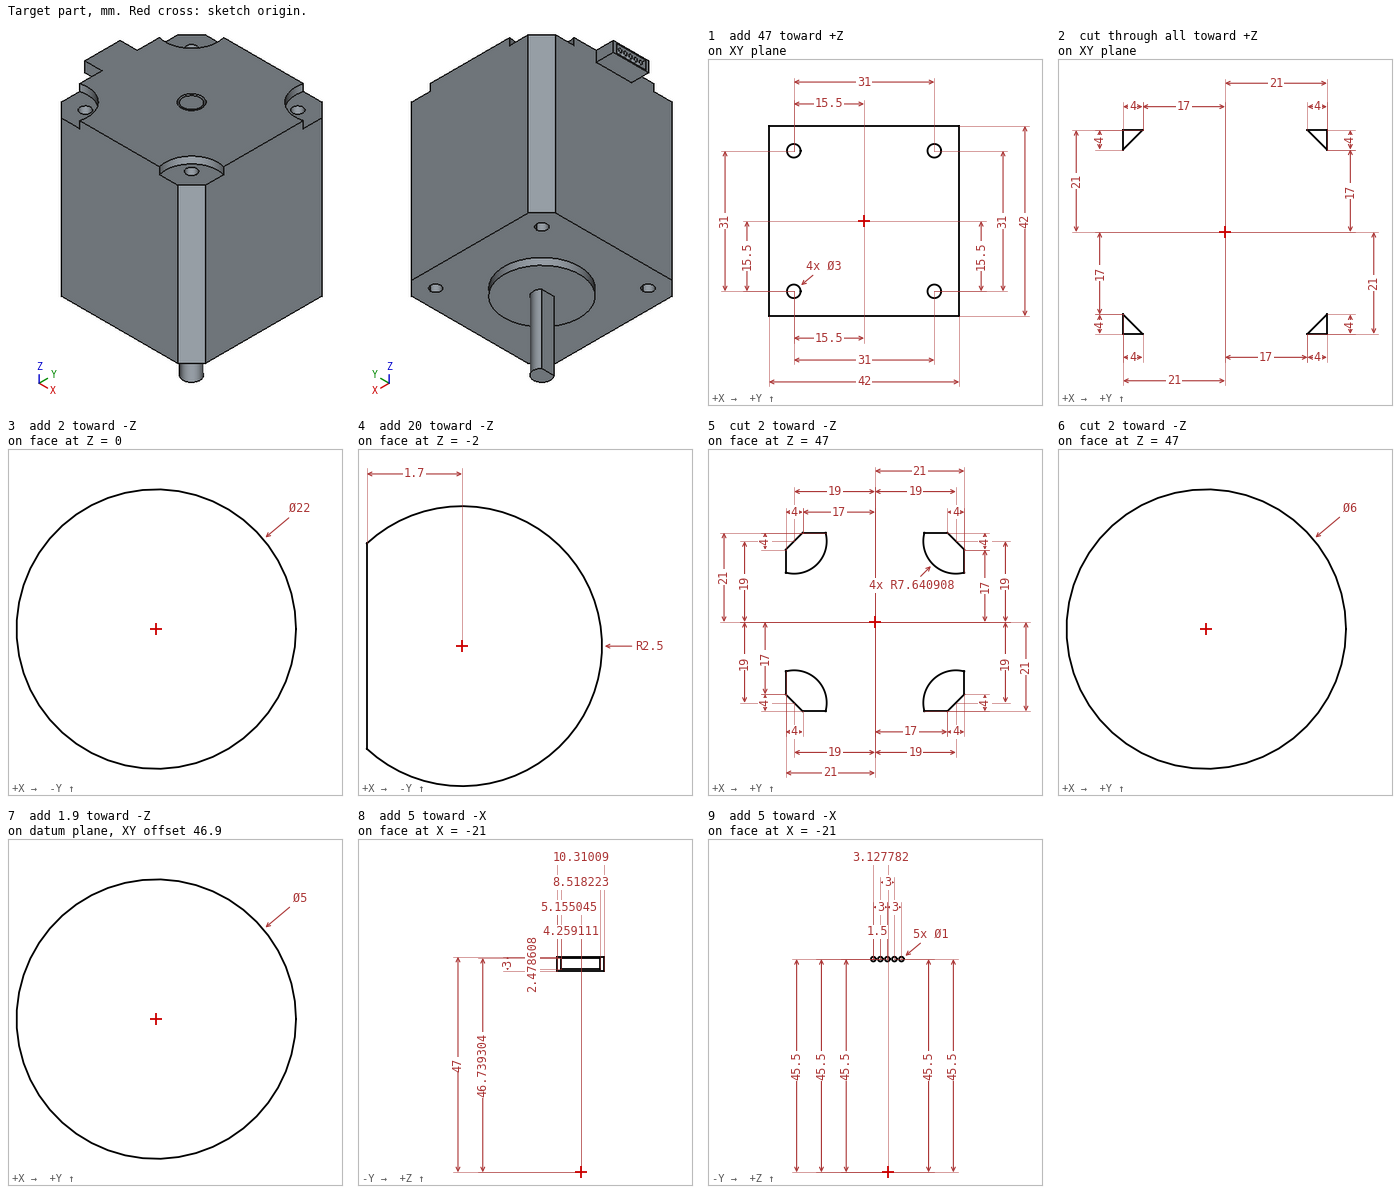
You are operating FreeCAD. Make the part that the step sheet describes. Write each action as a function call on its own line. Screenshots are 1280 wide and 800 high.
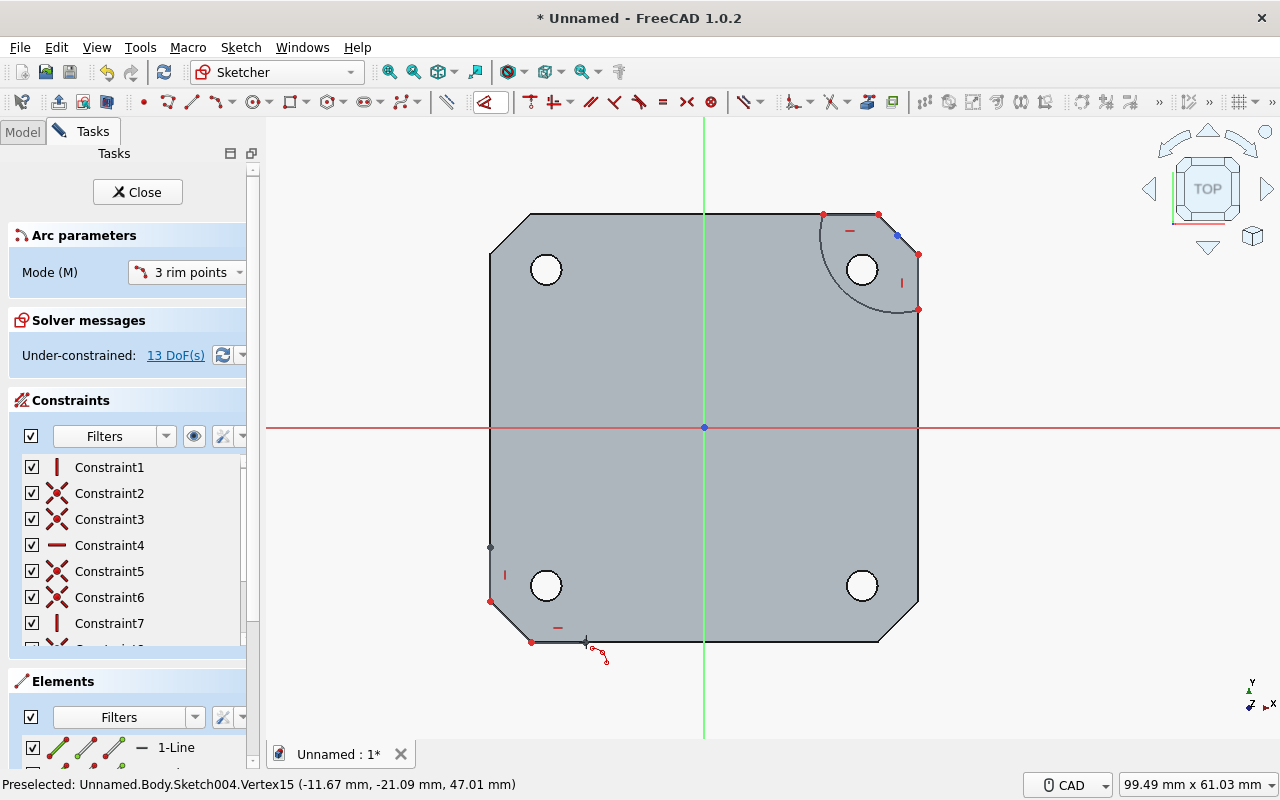
click(585, 643)
click(490, 547)
click(566, 566)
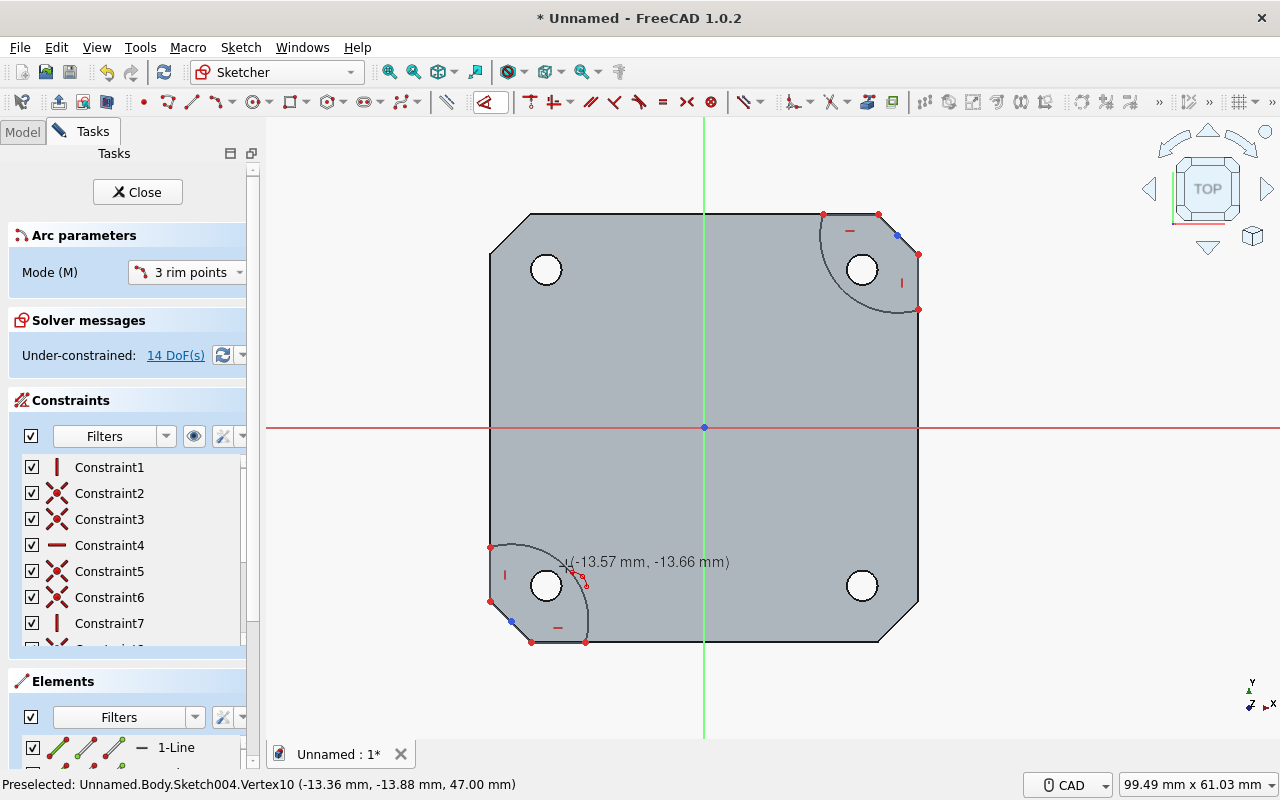
click(168, 102)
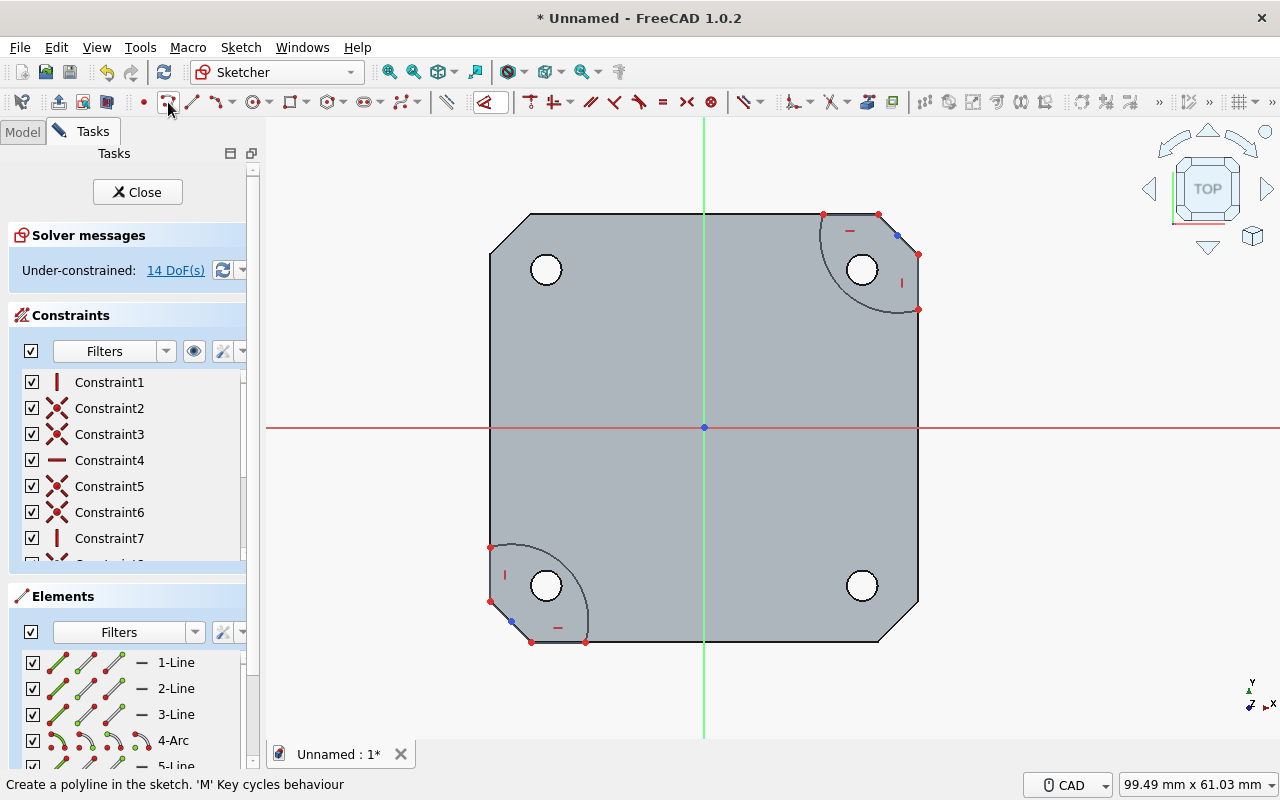
click(586, 214)
click(531, 214)
click(490, 254)
click(490, 309)
right_click(490, 309)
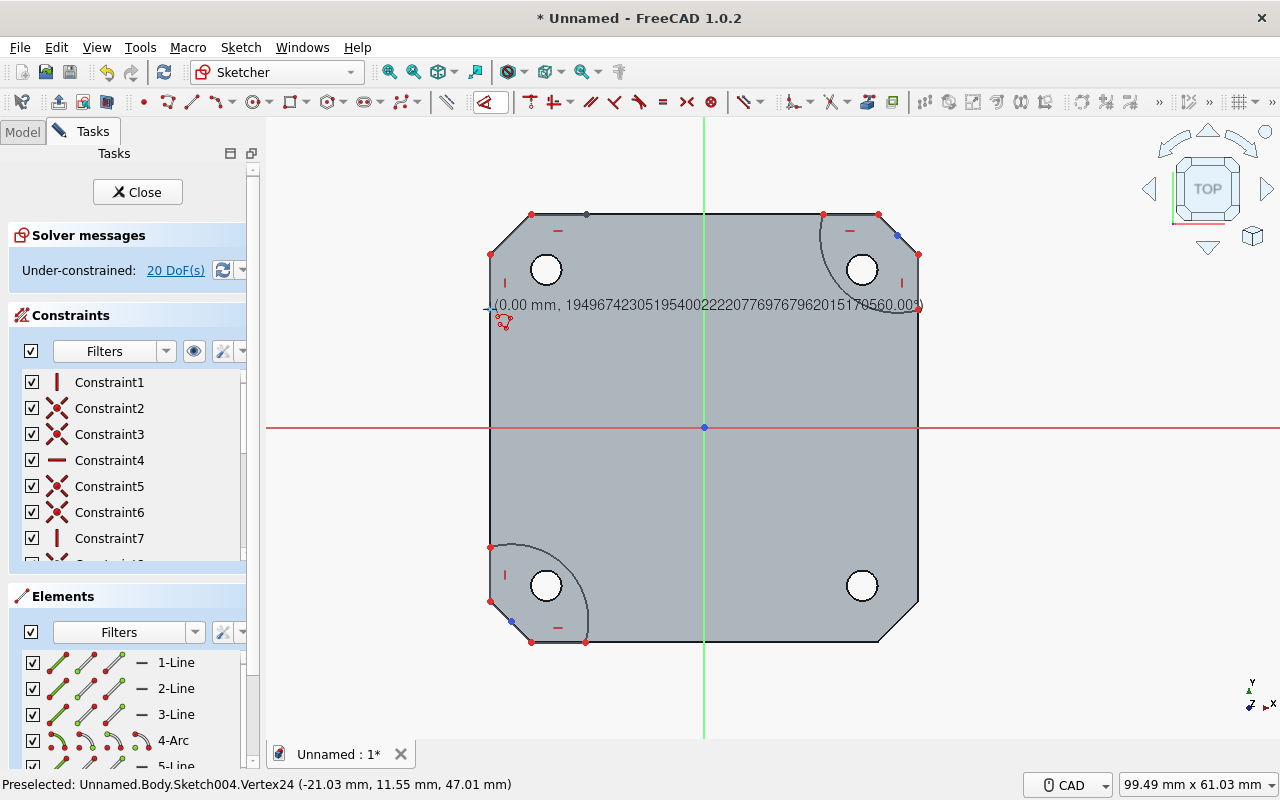
click(216, 102)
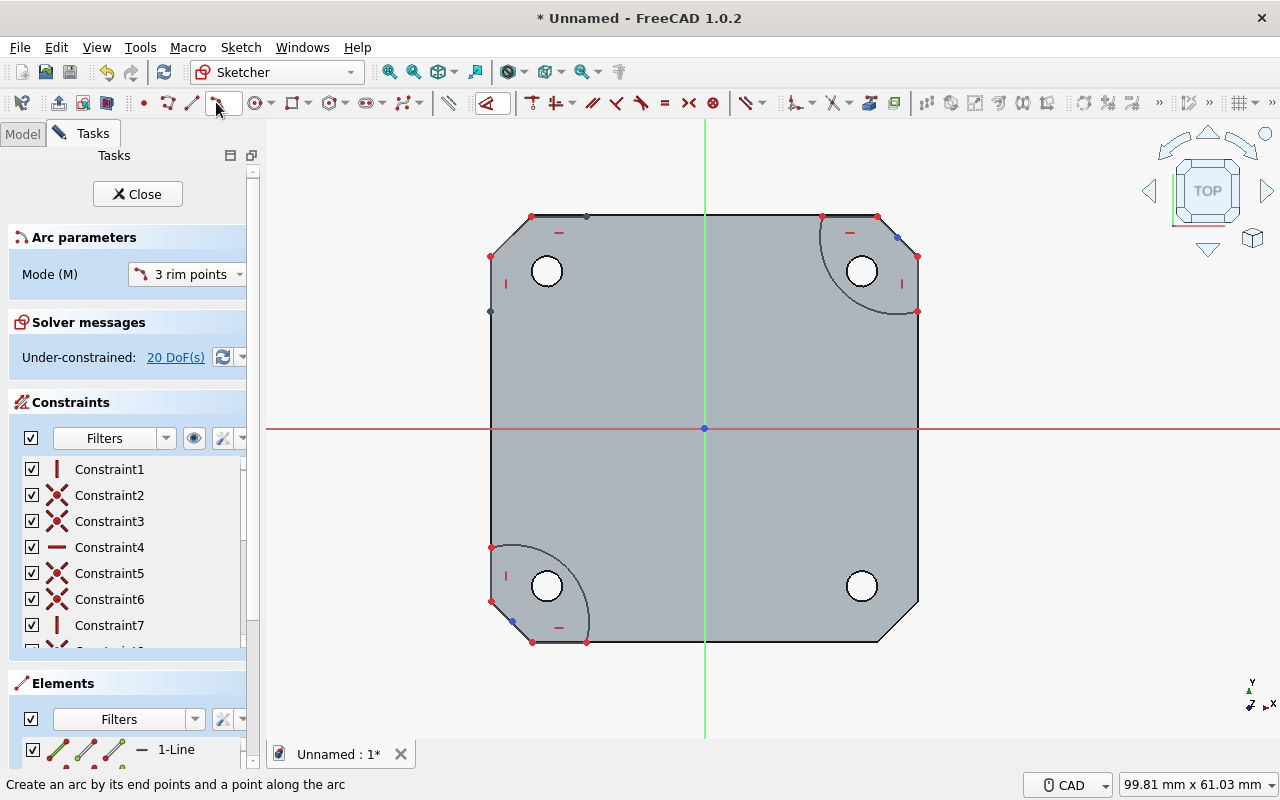
click(491, 311)
click(587, 217)
click(566, 291)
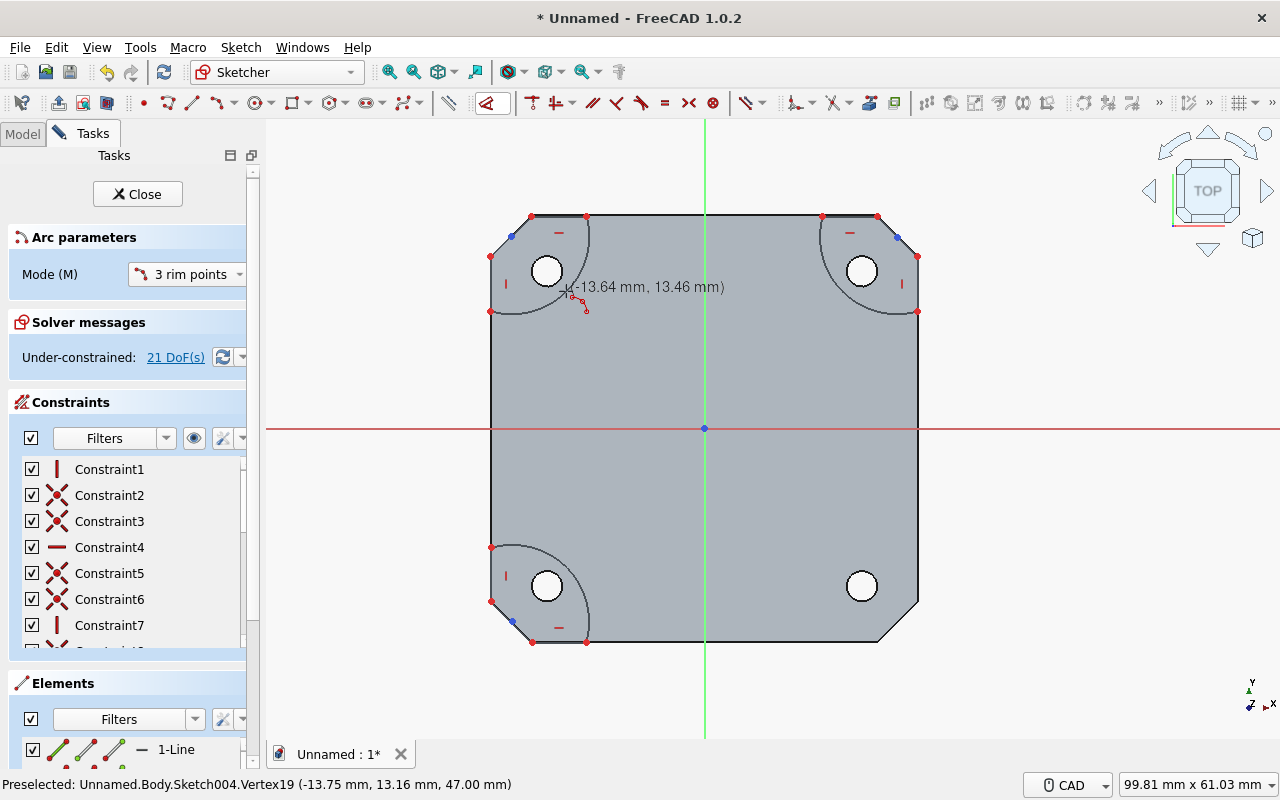
click(168, 104)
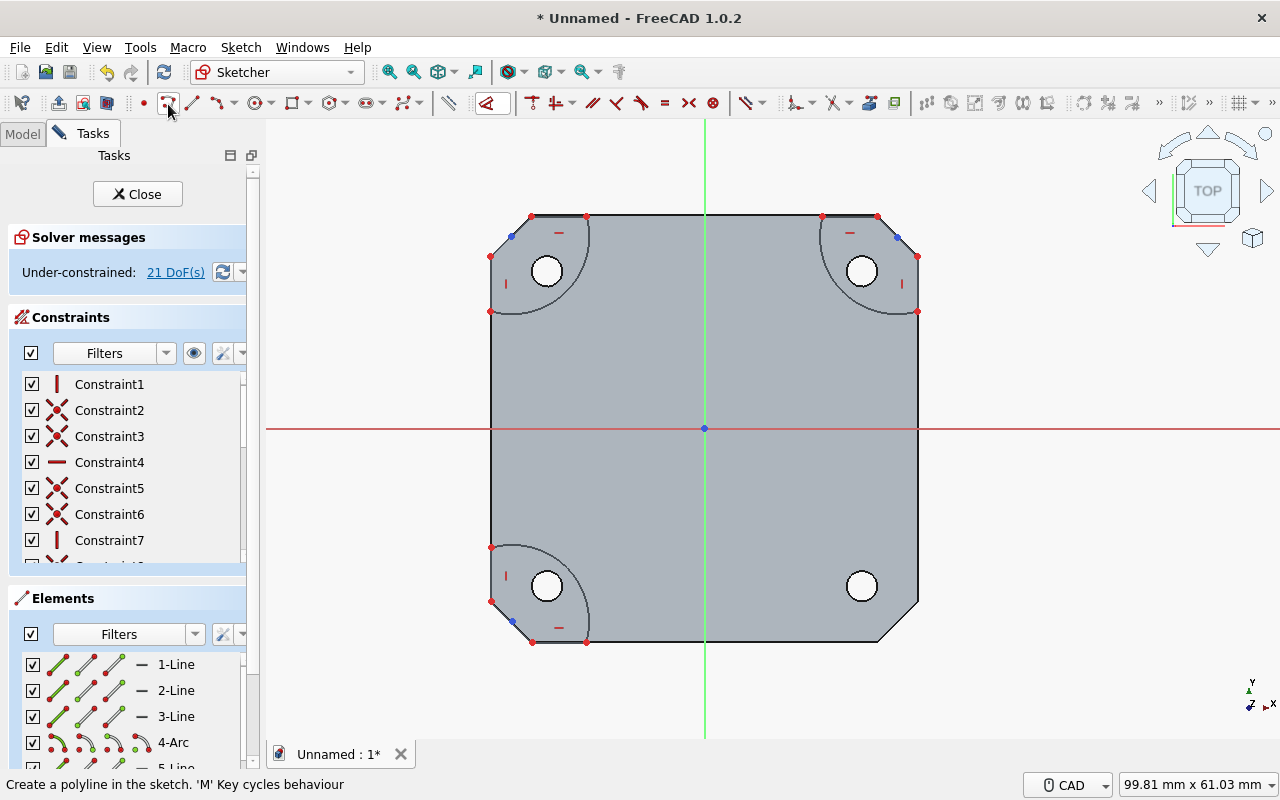
click(823, 642)
click(877, 642)
click(918, 601)
click(918, 547)
right_click(918, 547)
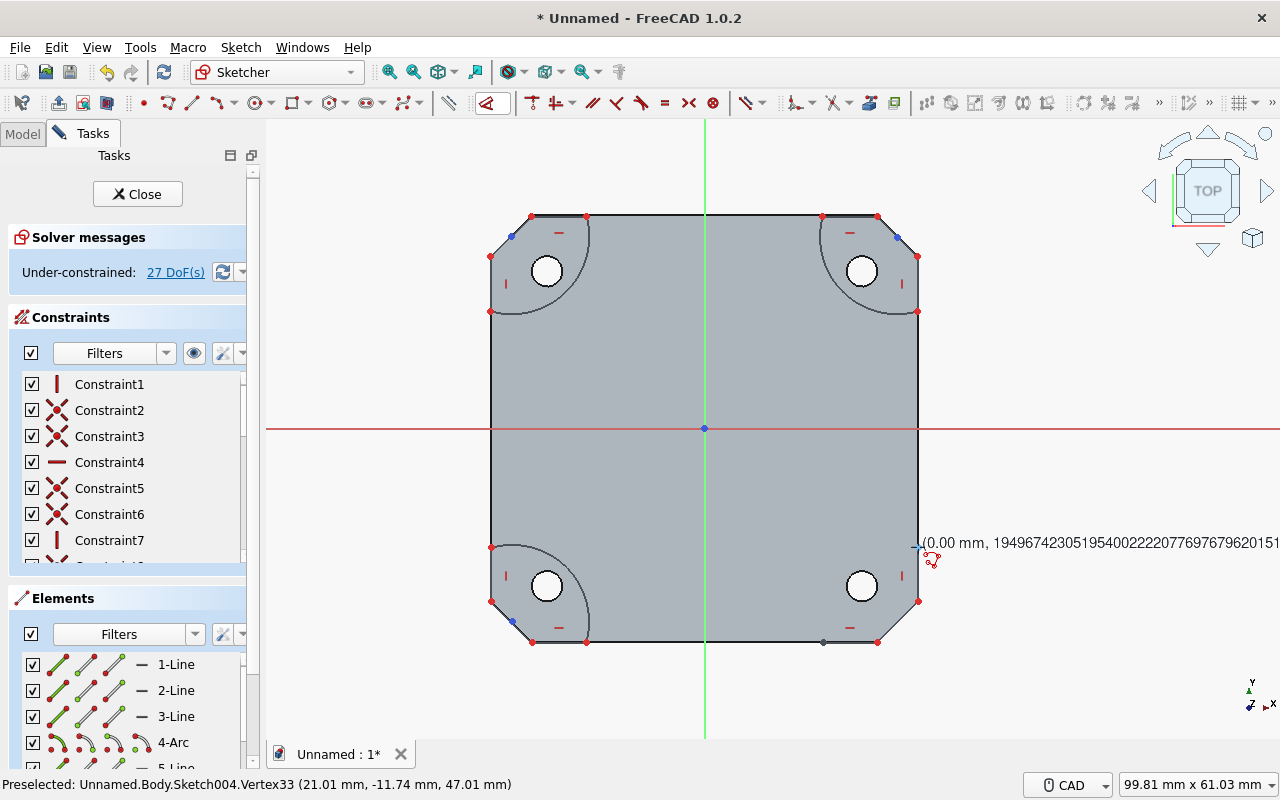
click(218, 104)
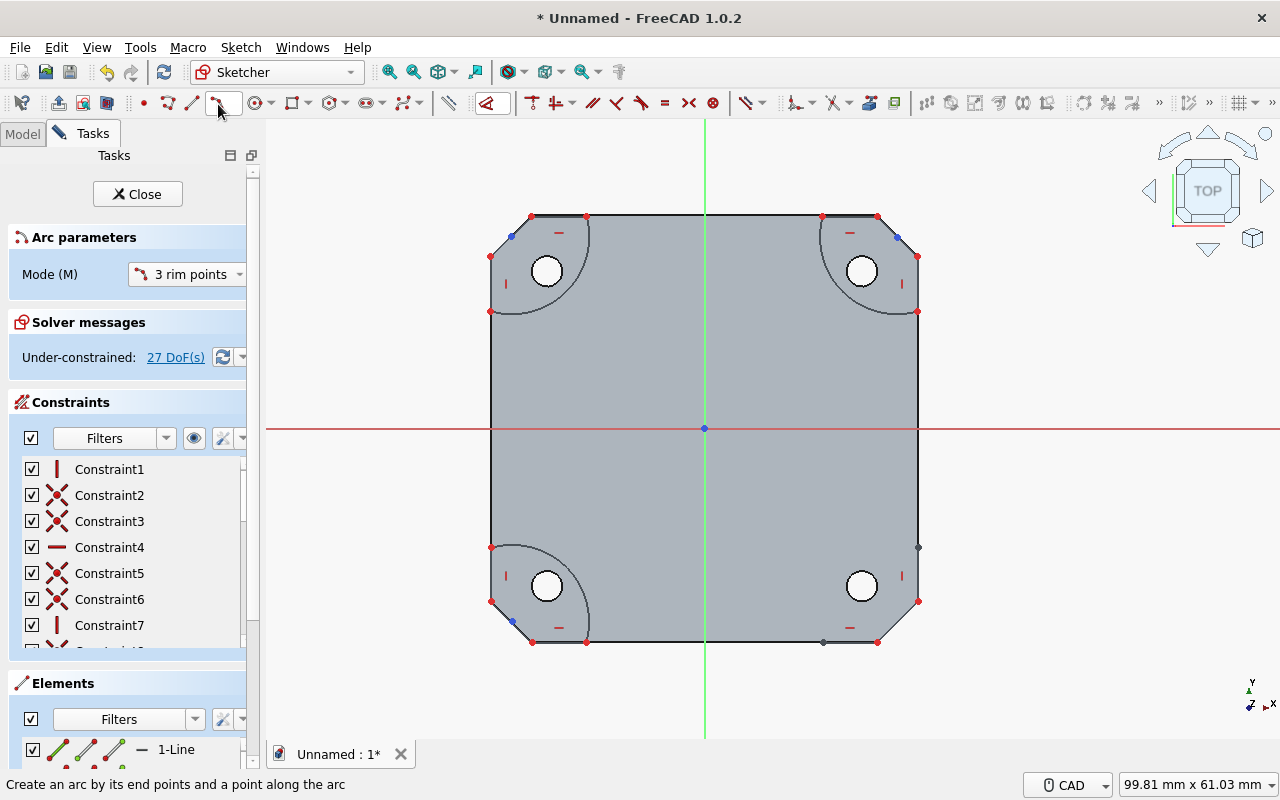
click(918, 548)
click(823, 643)
click(843, 567)
key(Escape)